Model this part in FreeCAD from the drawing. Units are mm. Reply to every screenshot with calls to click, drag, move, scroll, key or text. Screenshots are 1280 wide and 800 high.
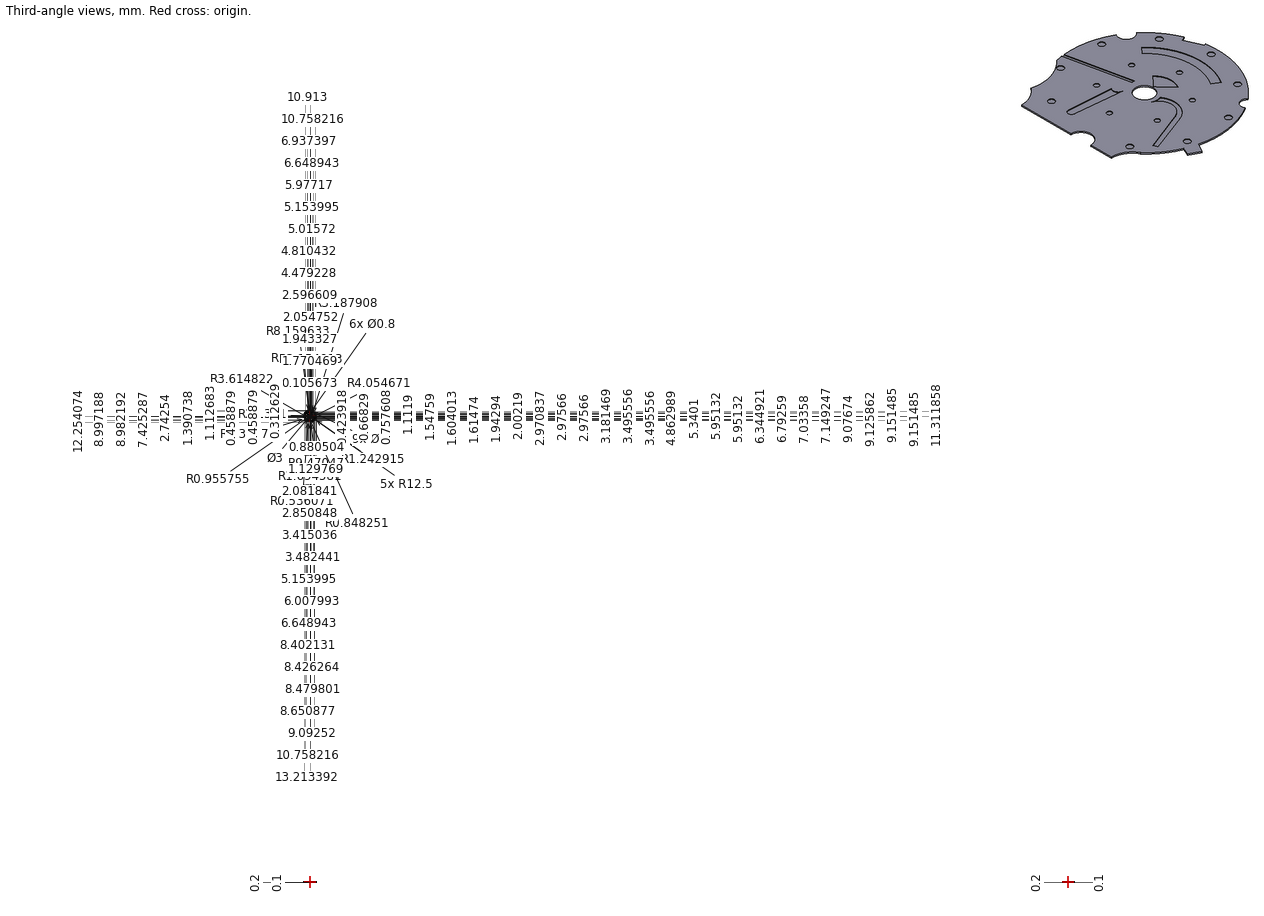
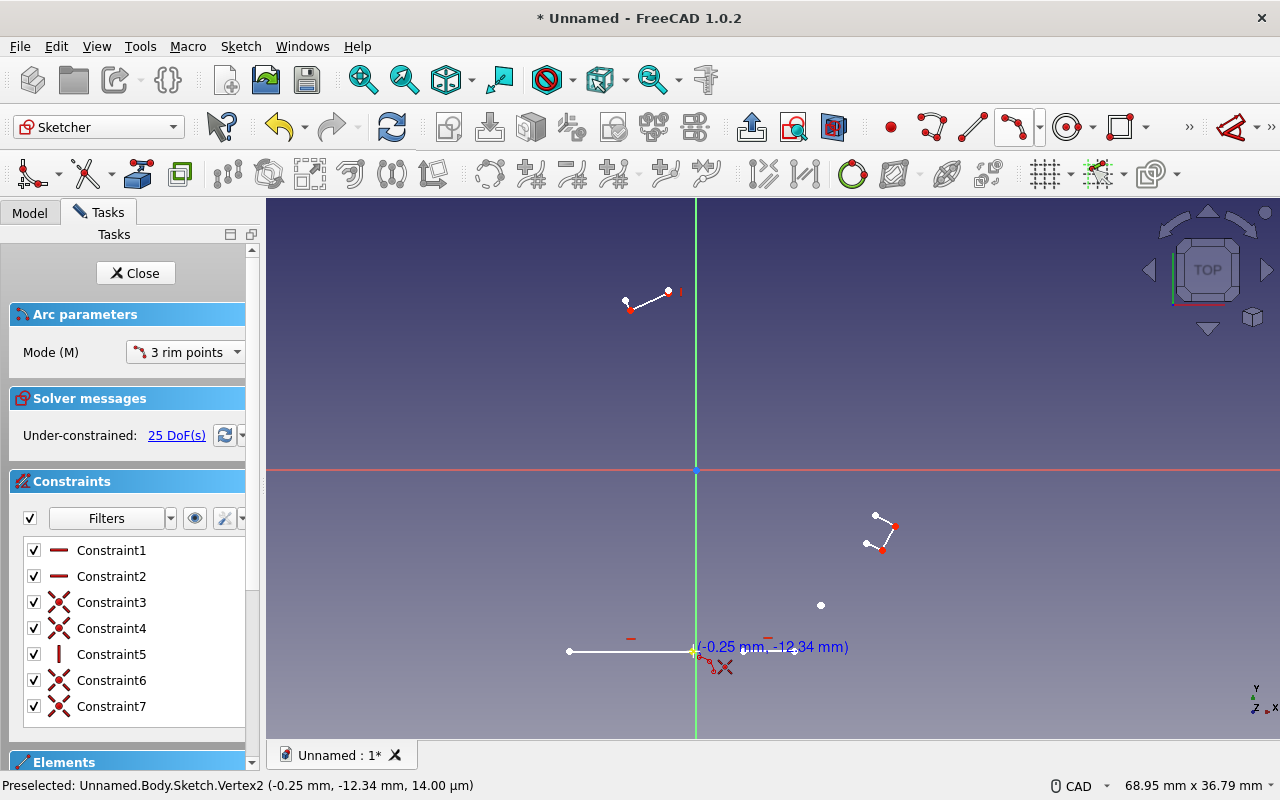
click(743, 651)
click(718, 625)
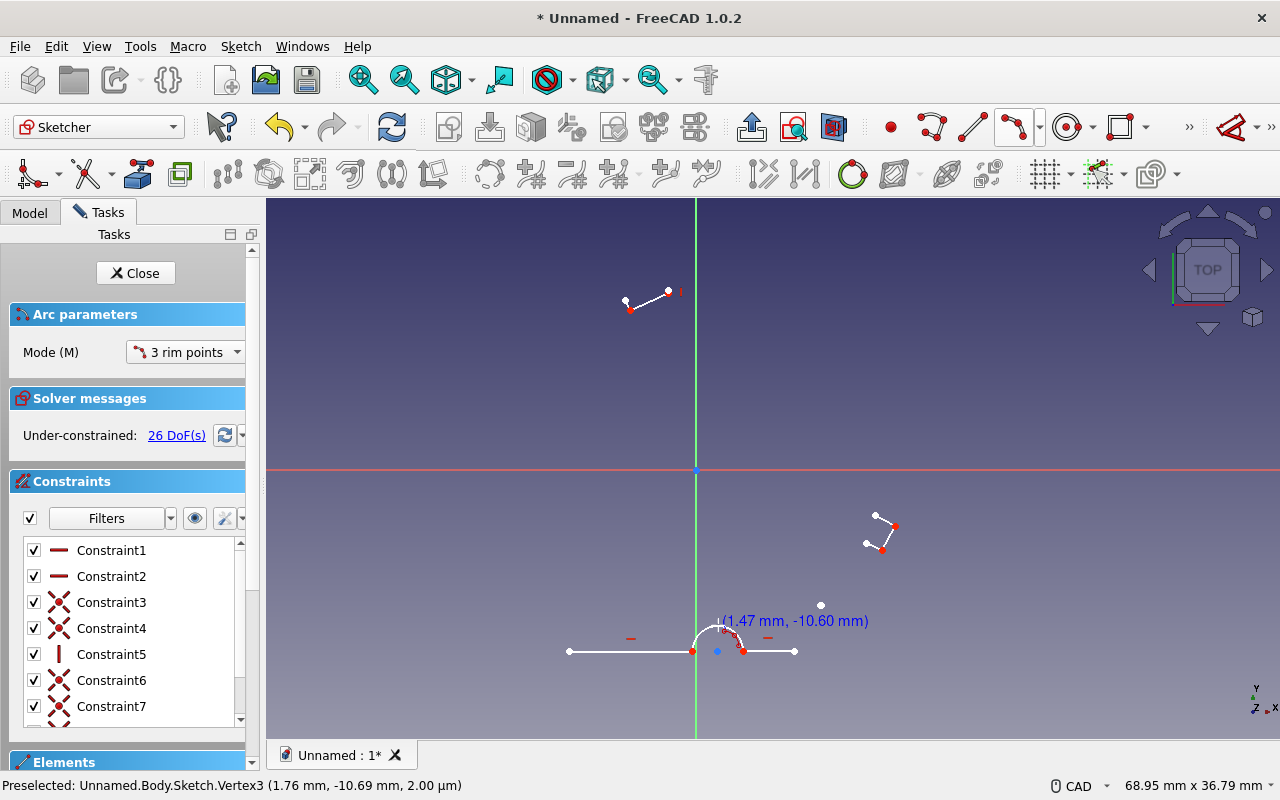
click(794, 651)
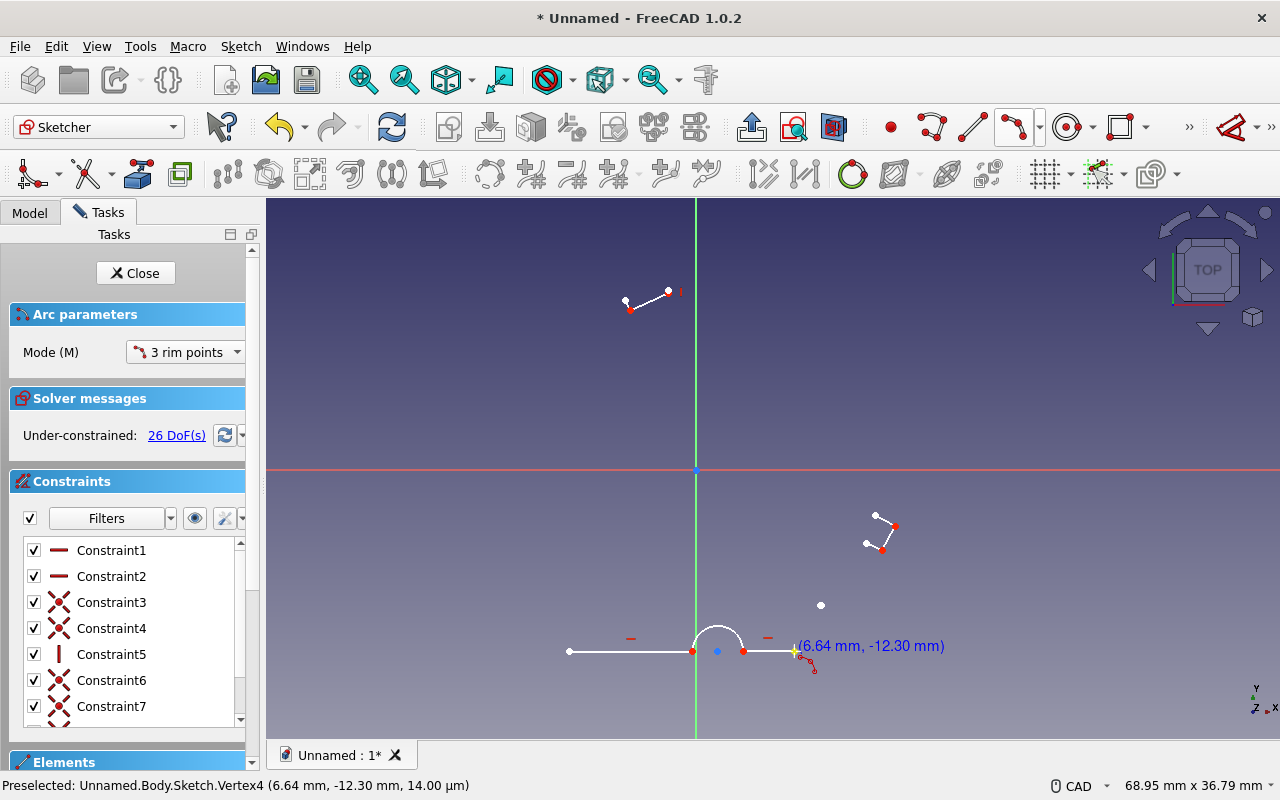
scroll(820, 604, up, 17)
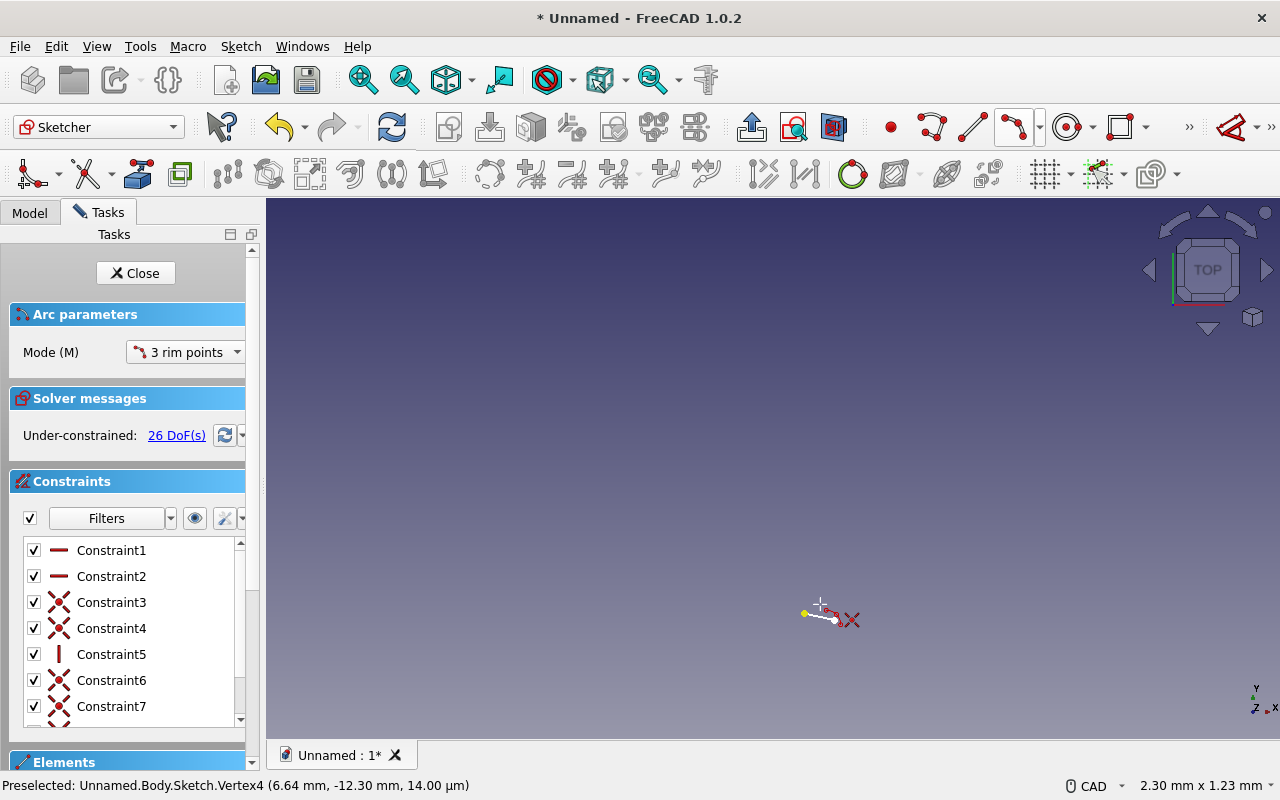
click(804, 584)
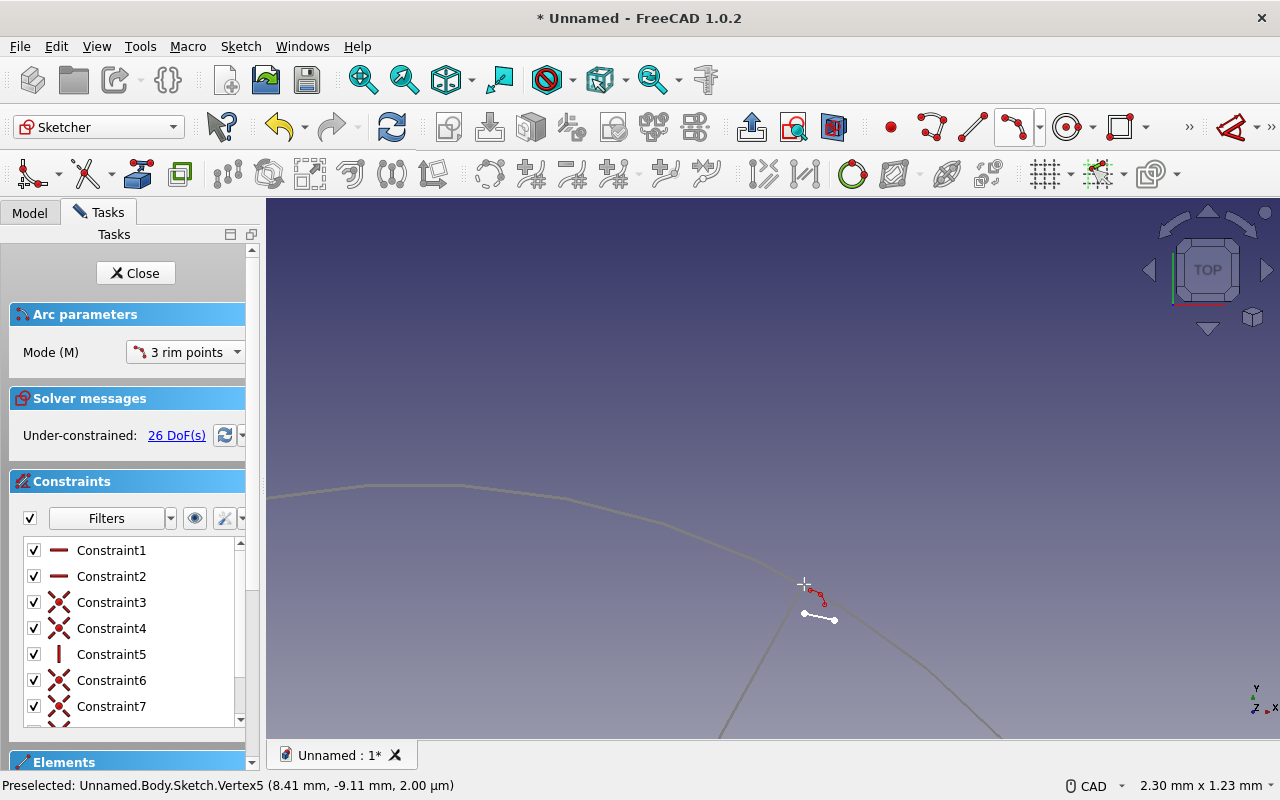
scroll(820, 604, down, 17)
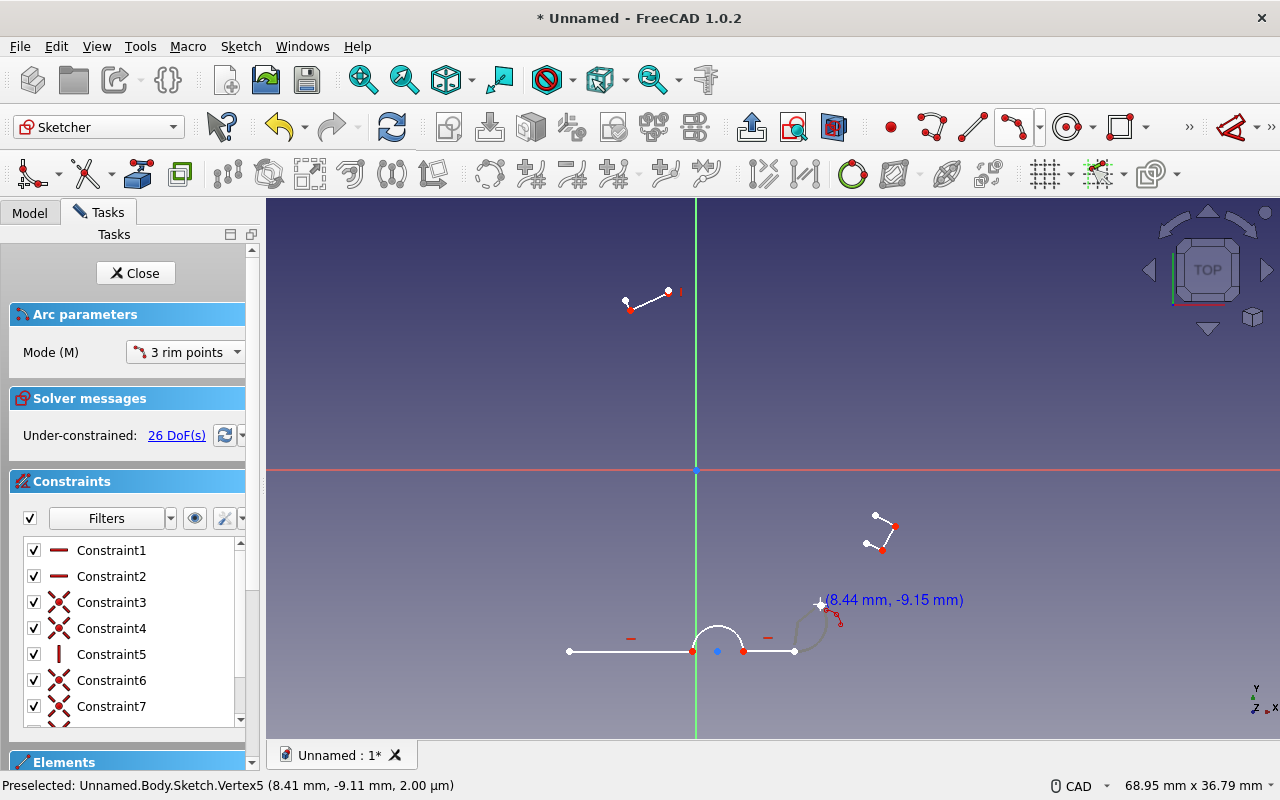
scroll(801, 624, up, 5)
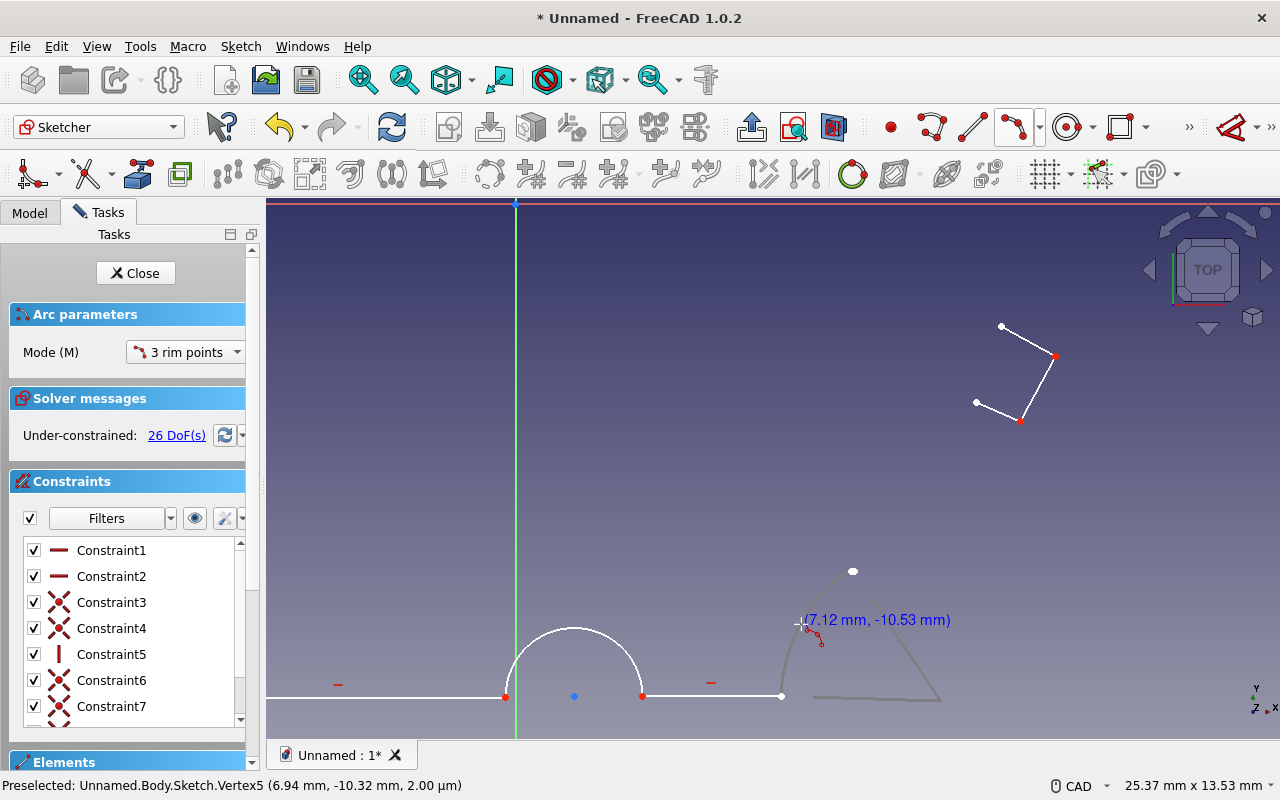
click(800, 622)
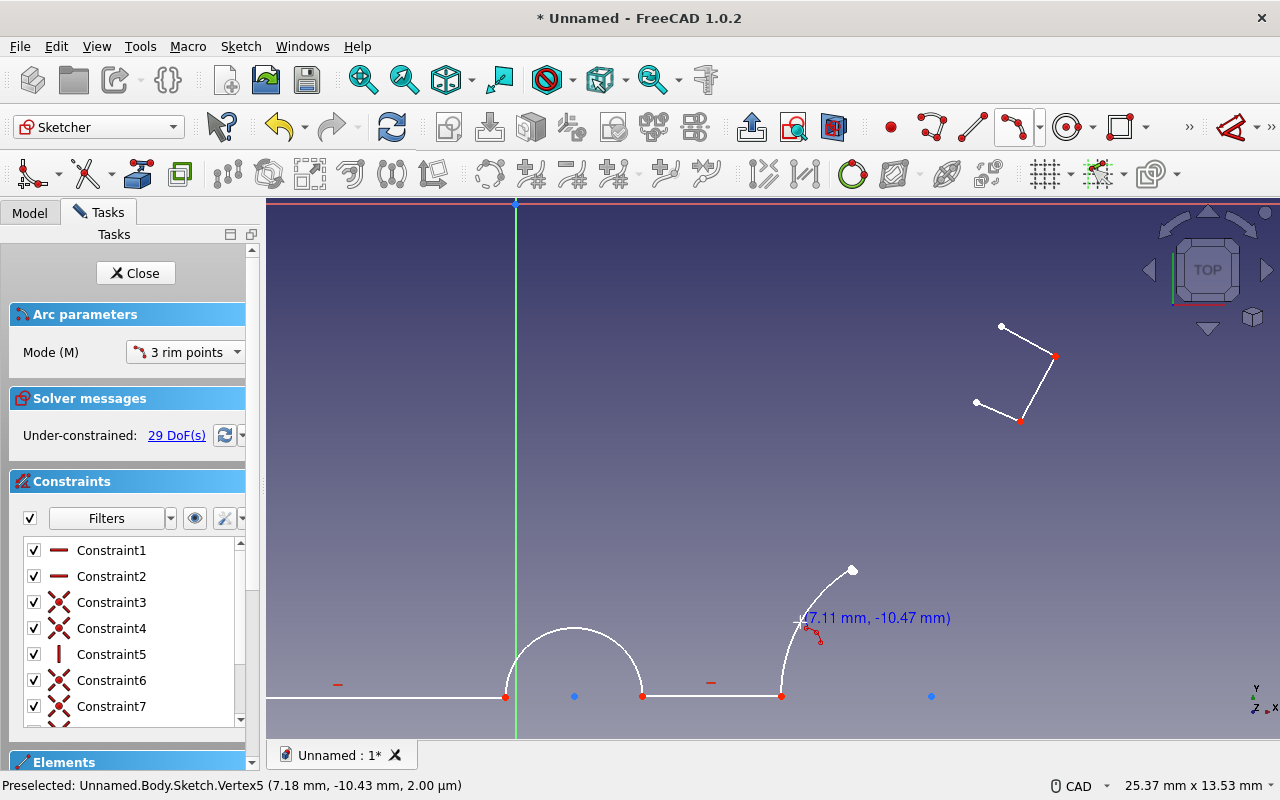
scroll(855, 572, up, 12)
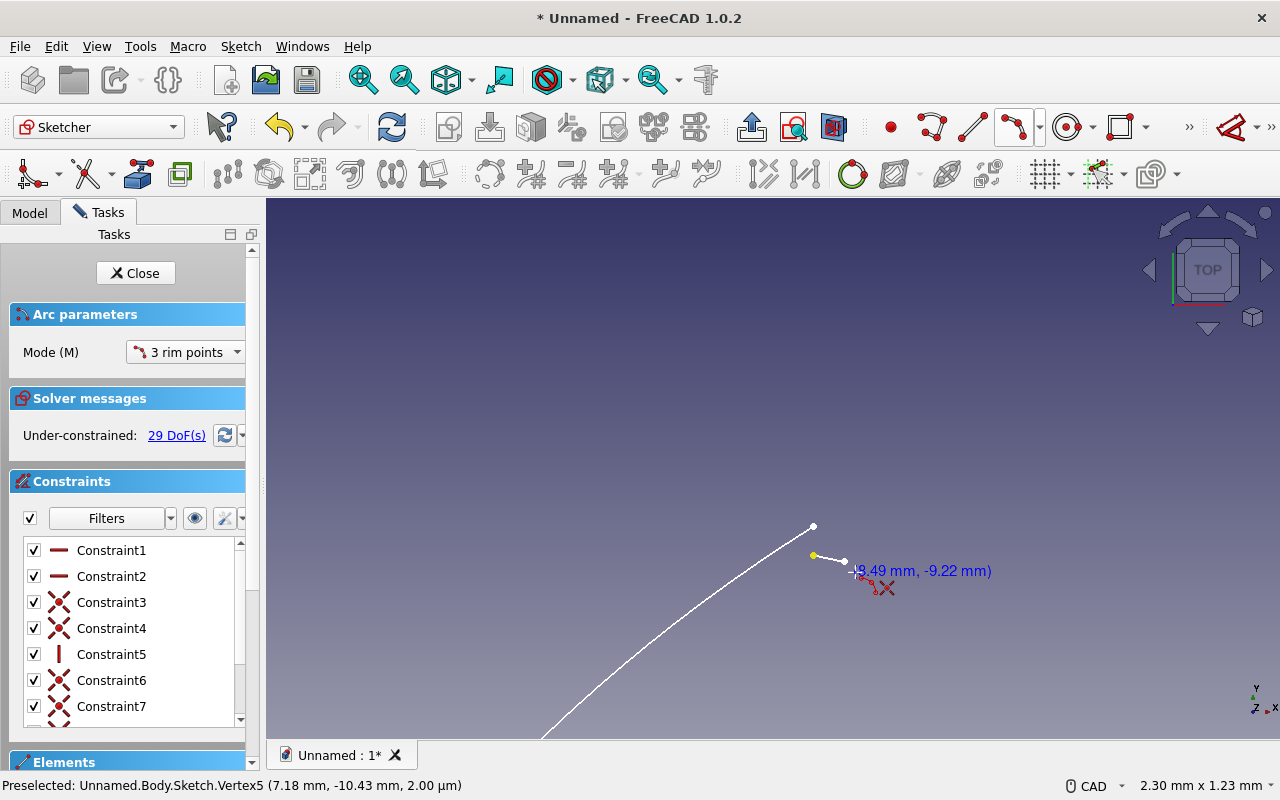
click(844, 562)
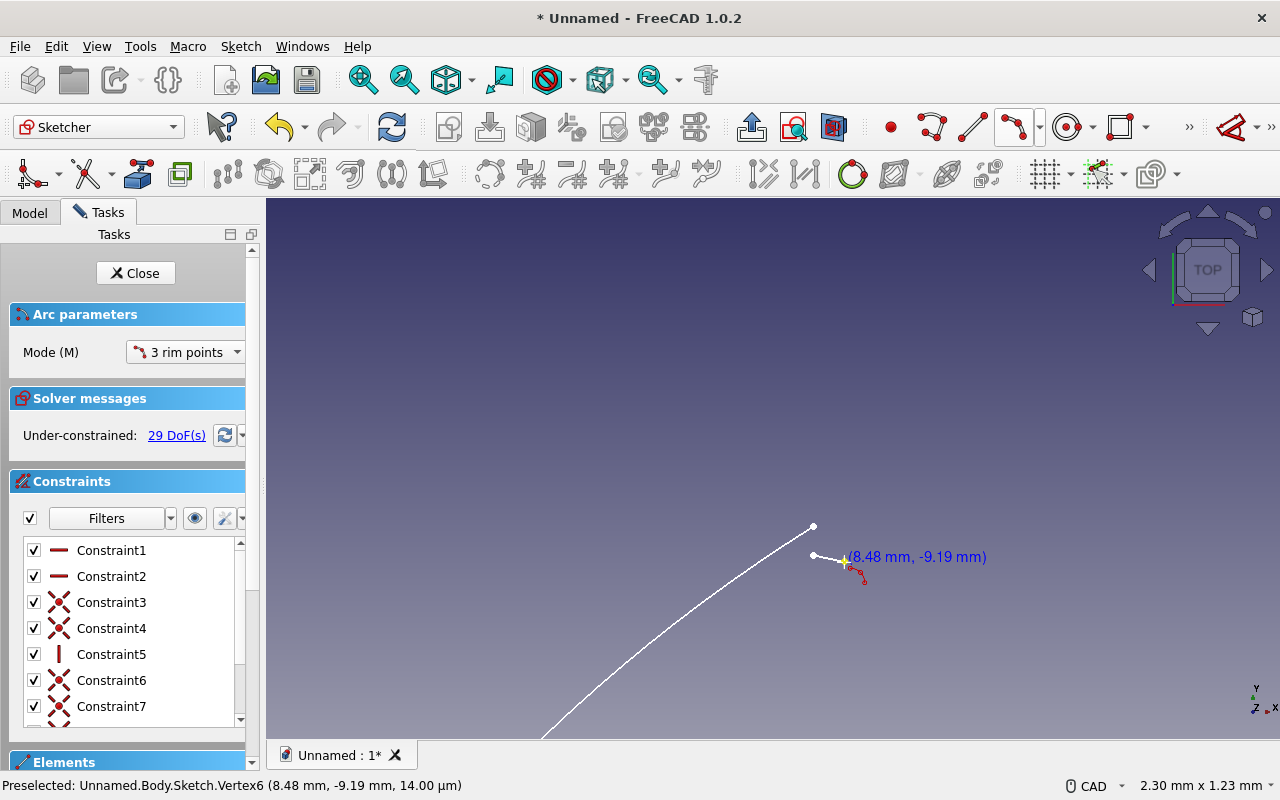
scroll(820, 606, down, 17)